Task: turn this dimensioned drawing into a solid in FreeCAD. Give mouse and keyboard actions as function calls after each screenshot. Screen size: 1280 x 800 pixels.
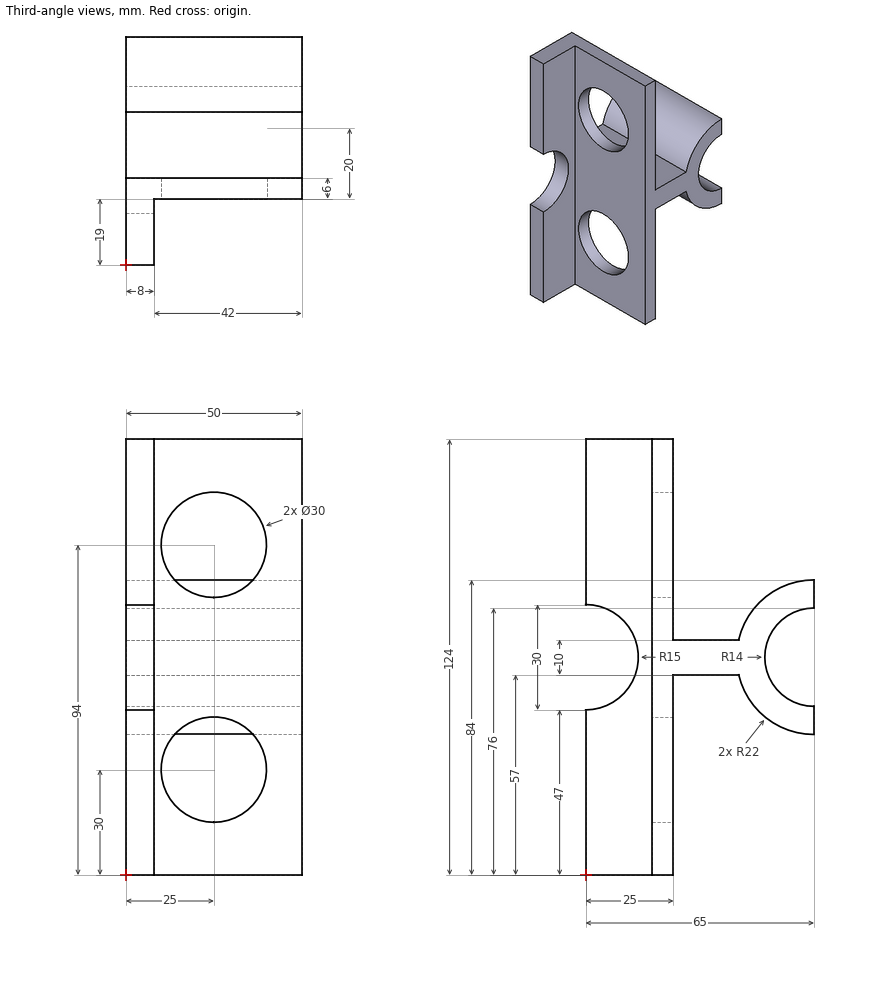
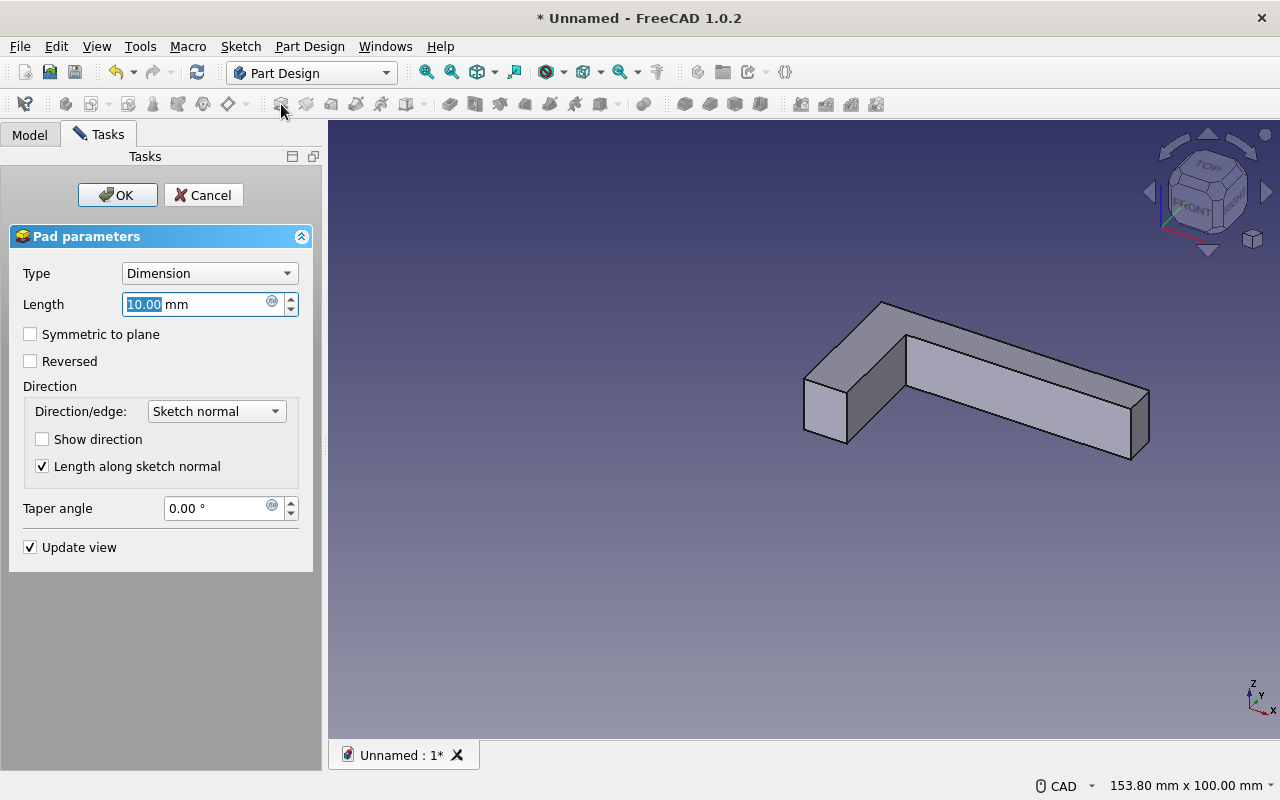
text(124)
key(Tab)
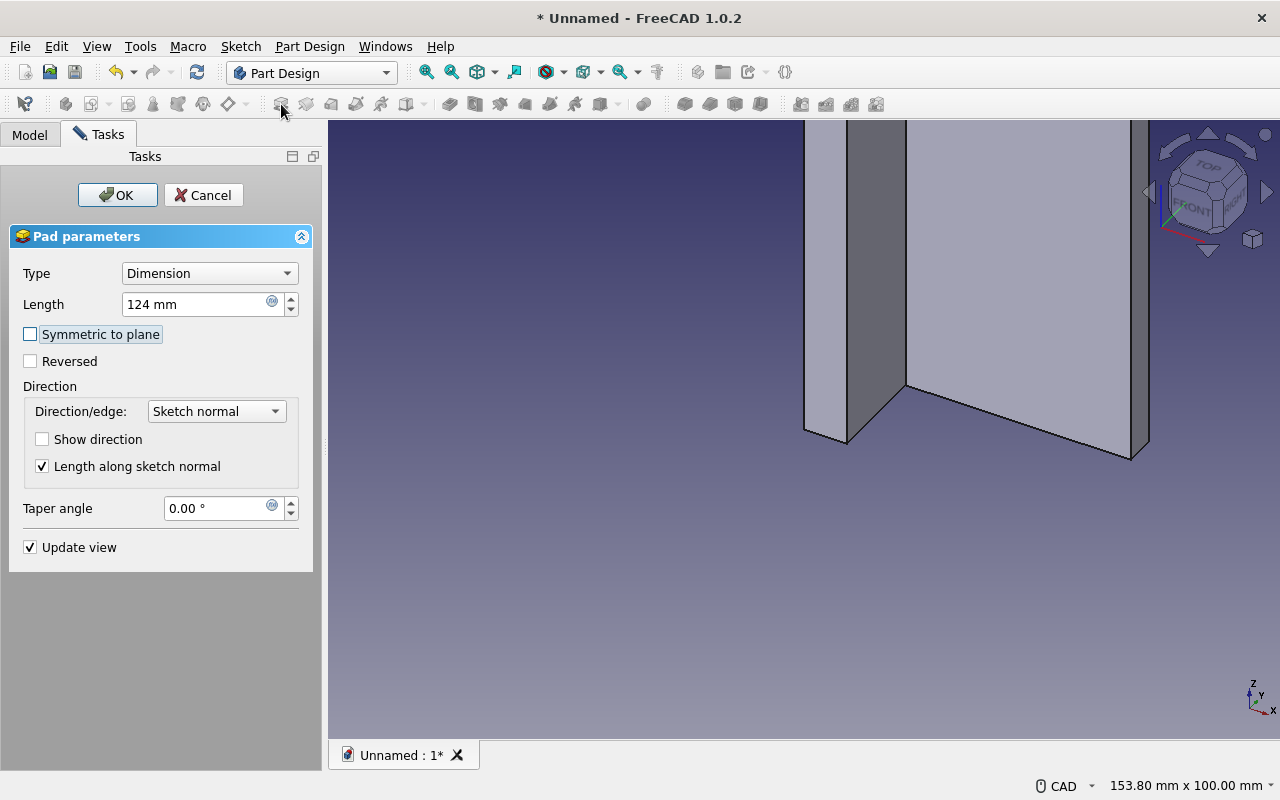
click(118, 195)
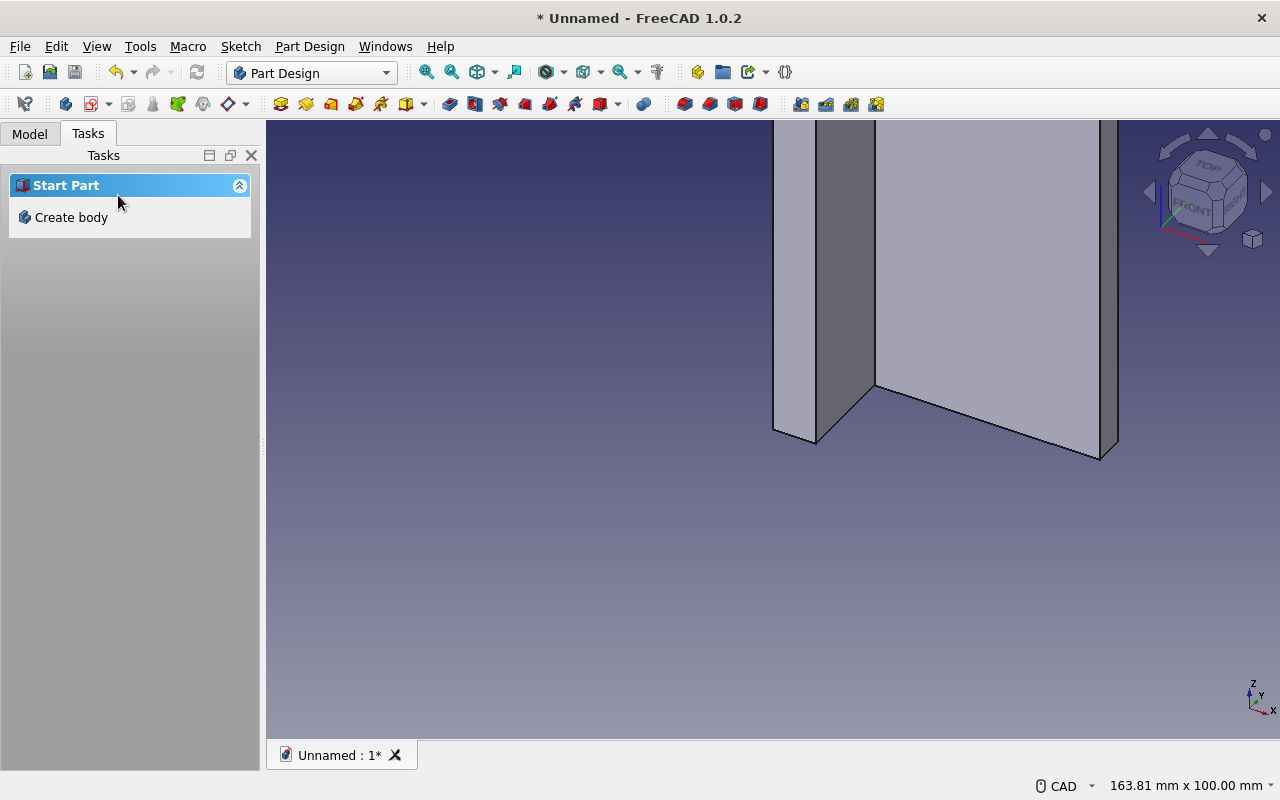
key(v)
key(f)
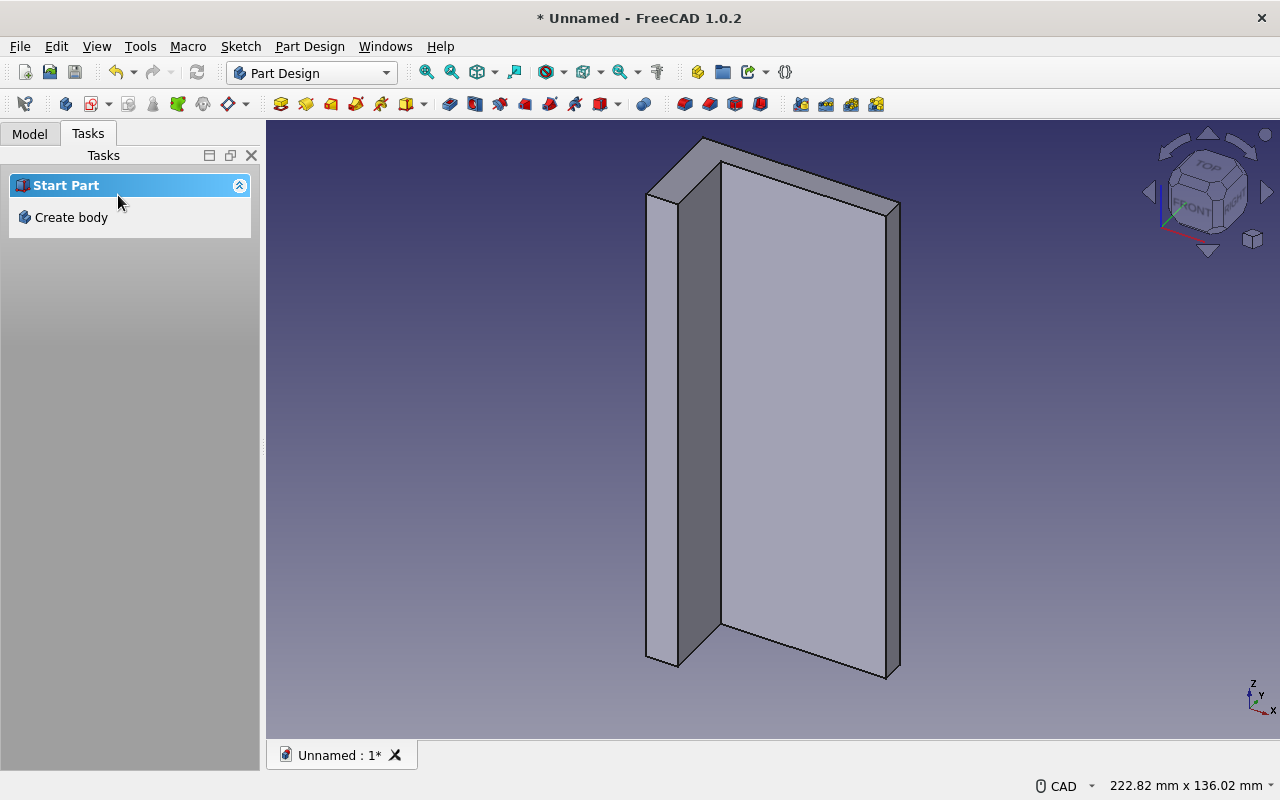
click(90, 104)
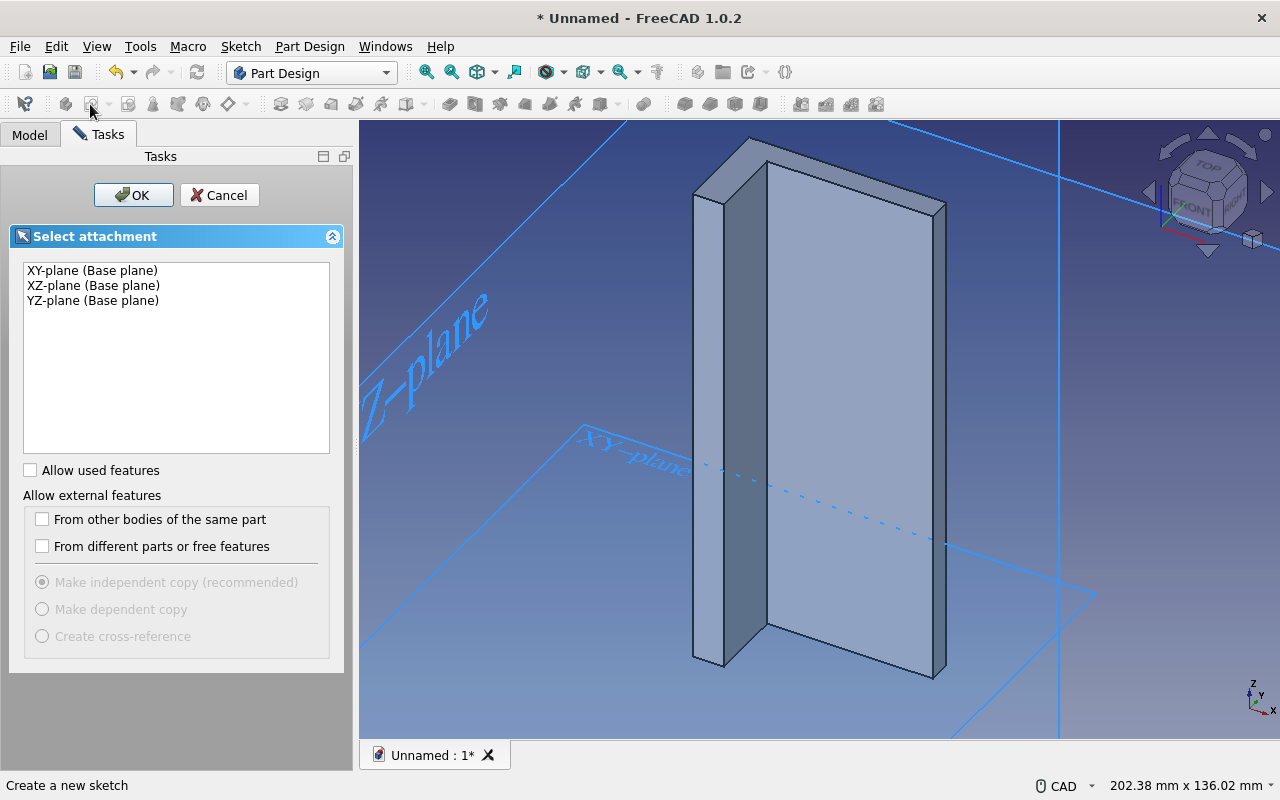
click(84, 300)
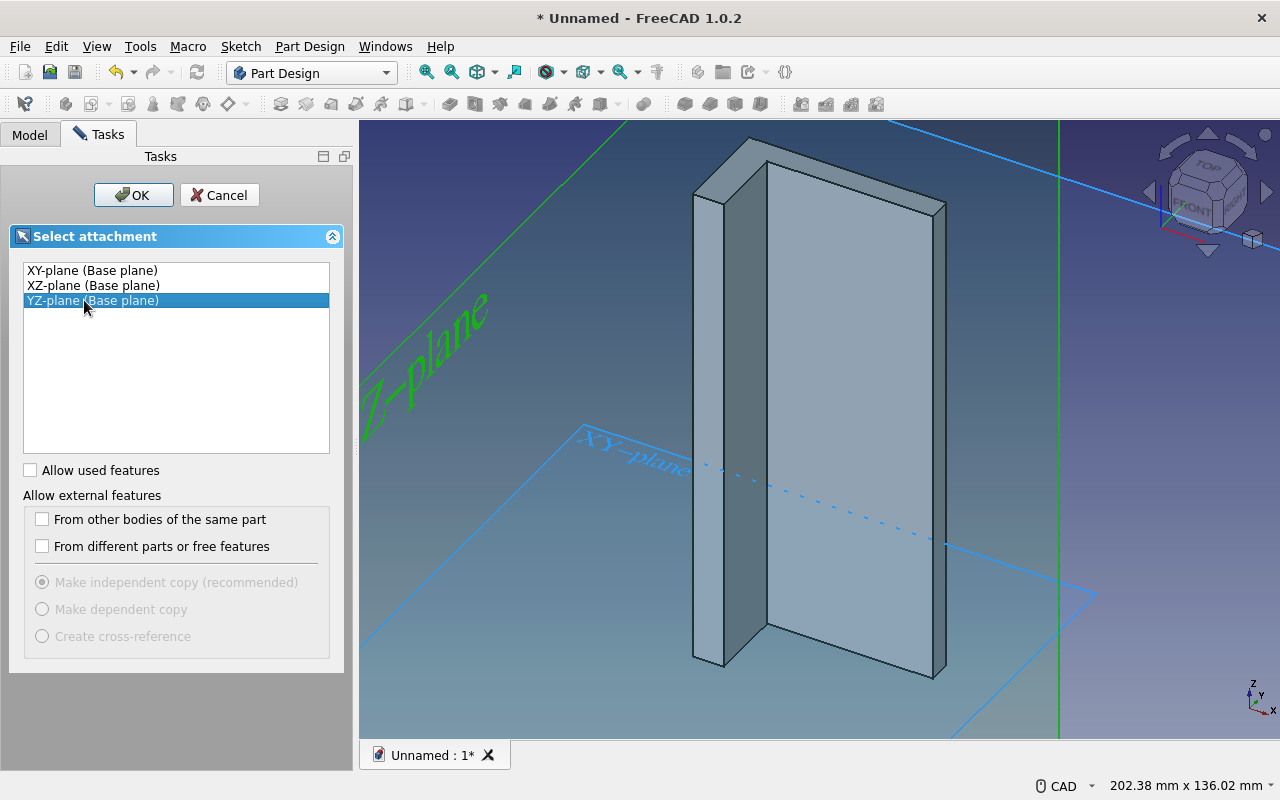
click(134, 195)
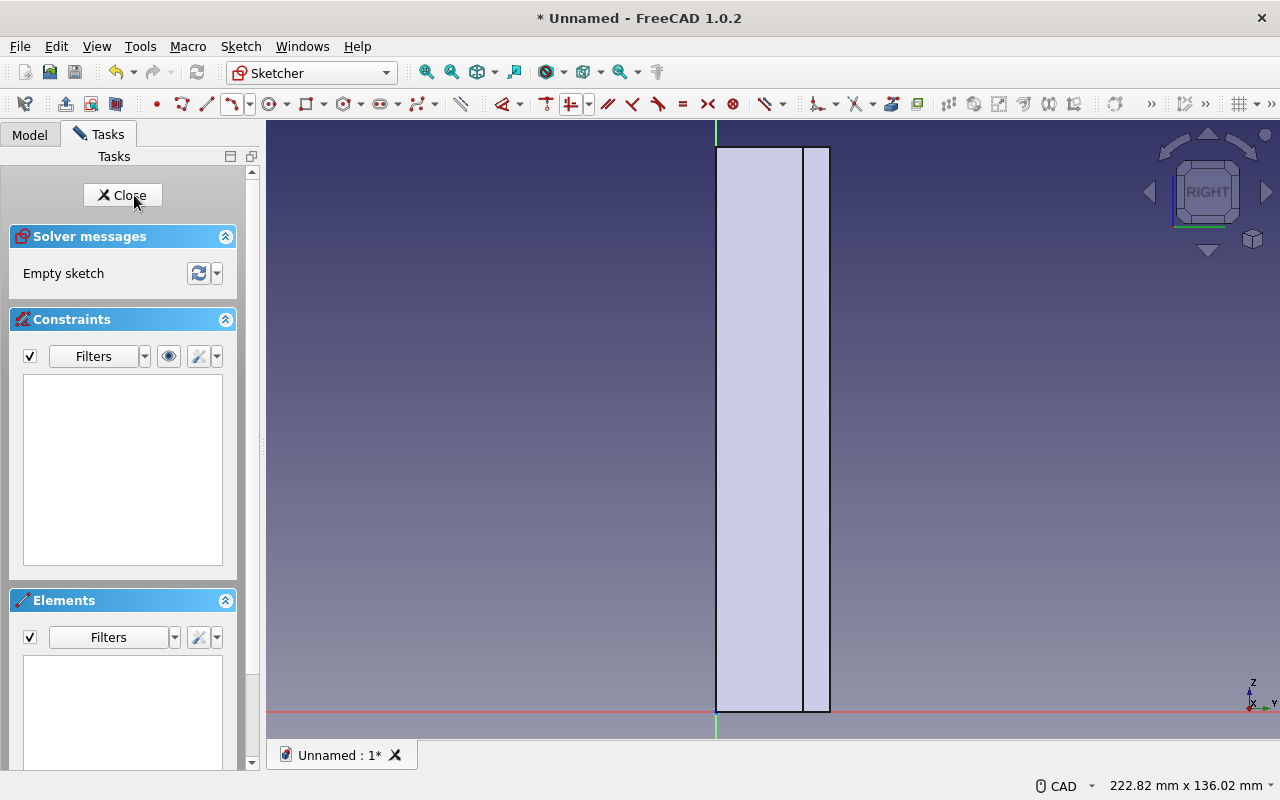
key(q)
key(s)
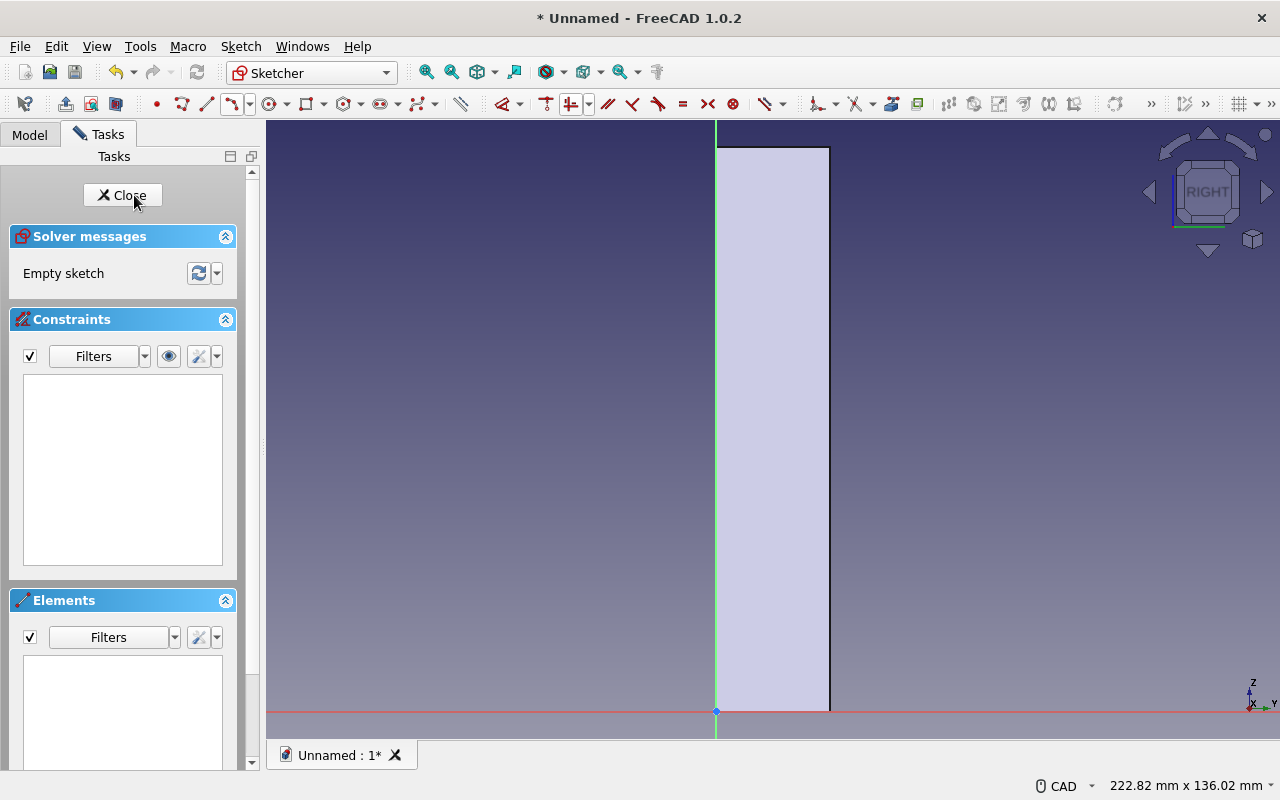
scroll(294, 148, down, 1)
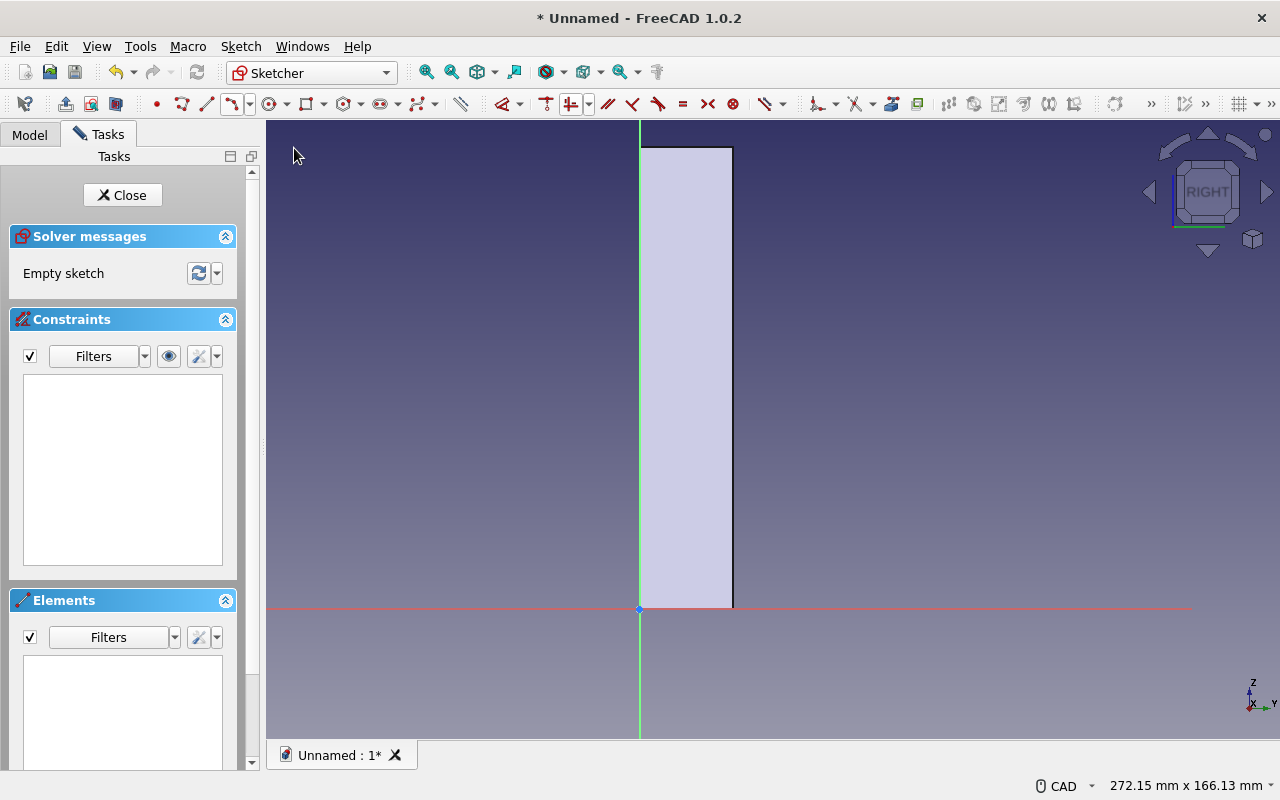
click(207, 104)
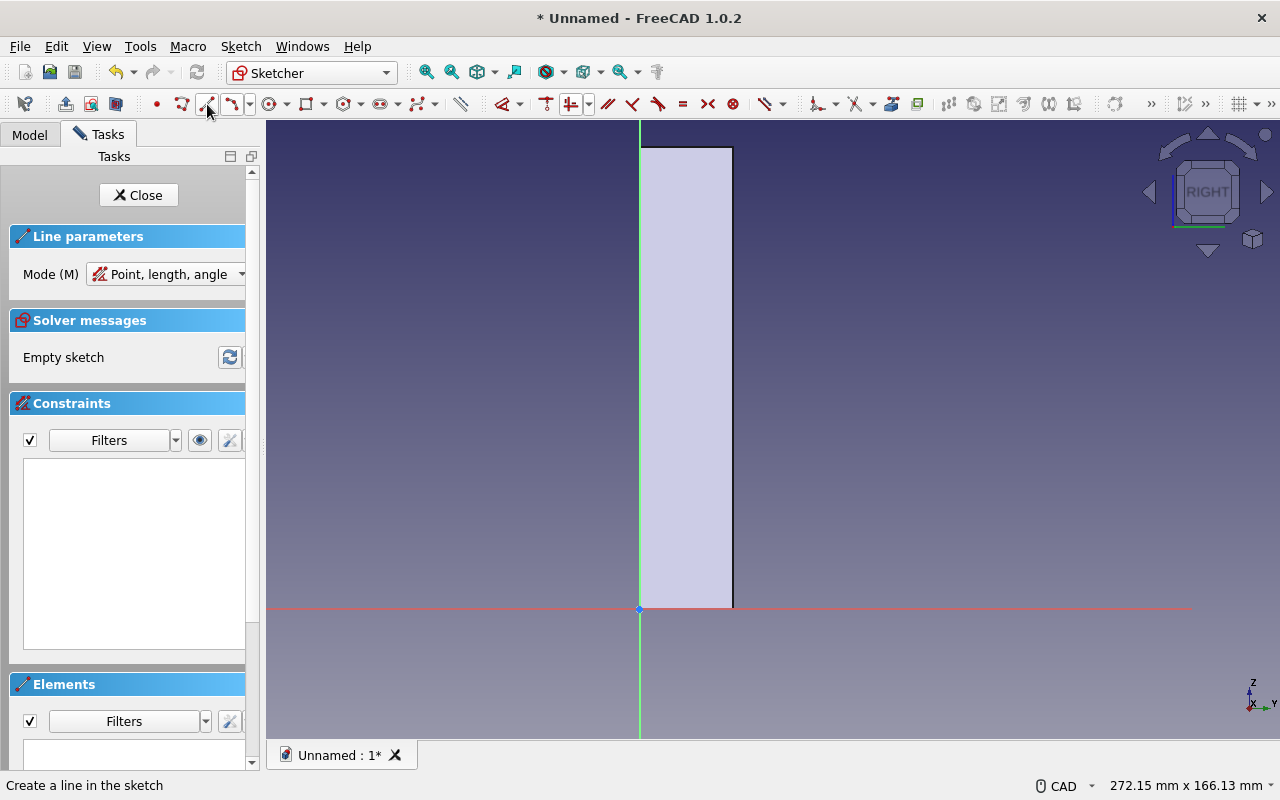
click(882, 297)
click(882, 460)